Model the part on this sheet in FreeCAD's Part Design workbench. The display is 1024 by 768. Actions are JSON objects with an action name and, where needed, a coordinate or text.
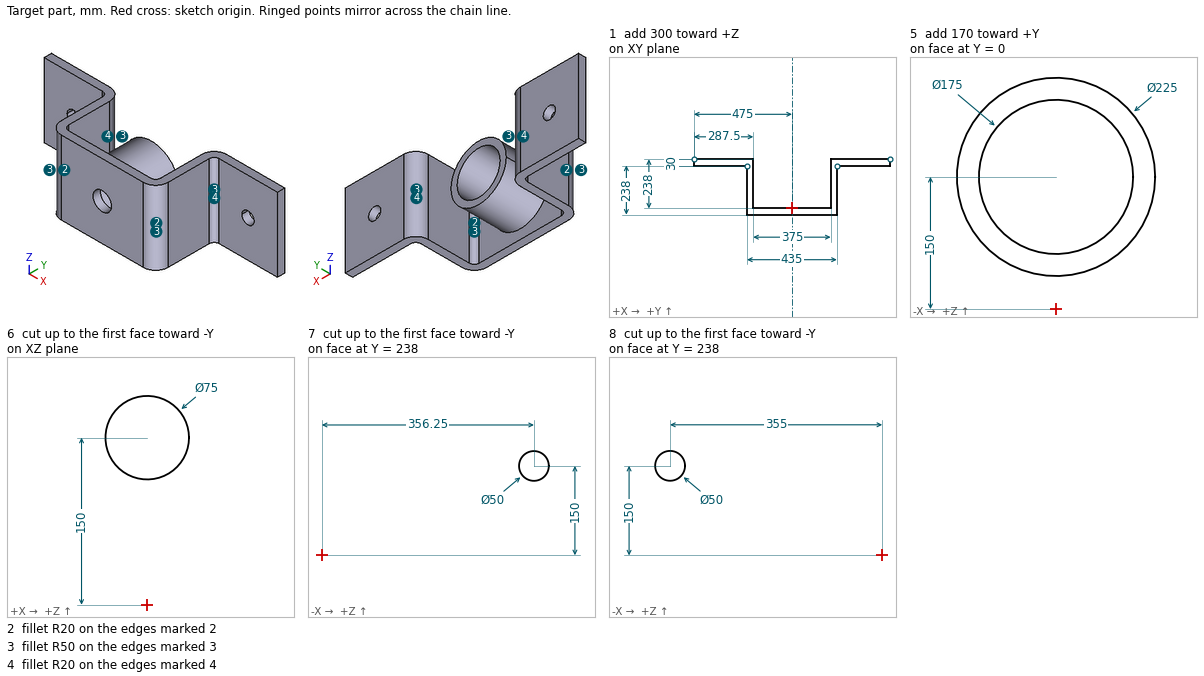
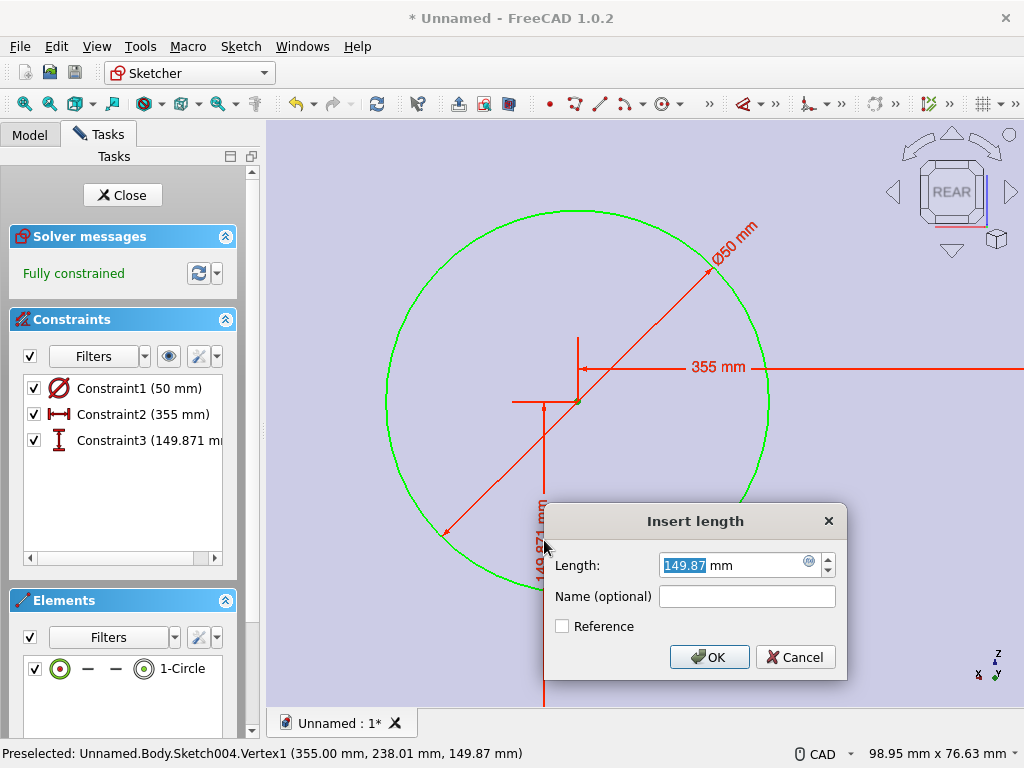
{"action": "type", "text": "150"}
{"action": "key", "text": "Return"}
{"action": "key", "text": "Escape"}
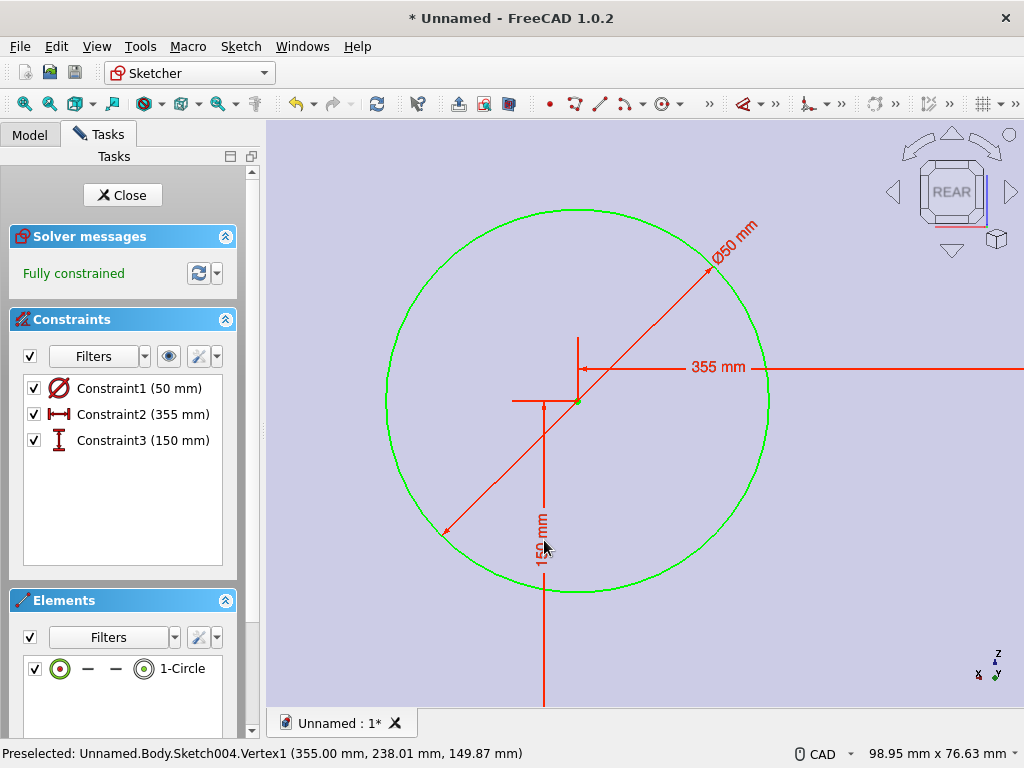
{"action": "left_click", "coordinate": [123, 195]}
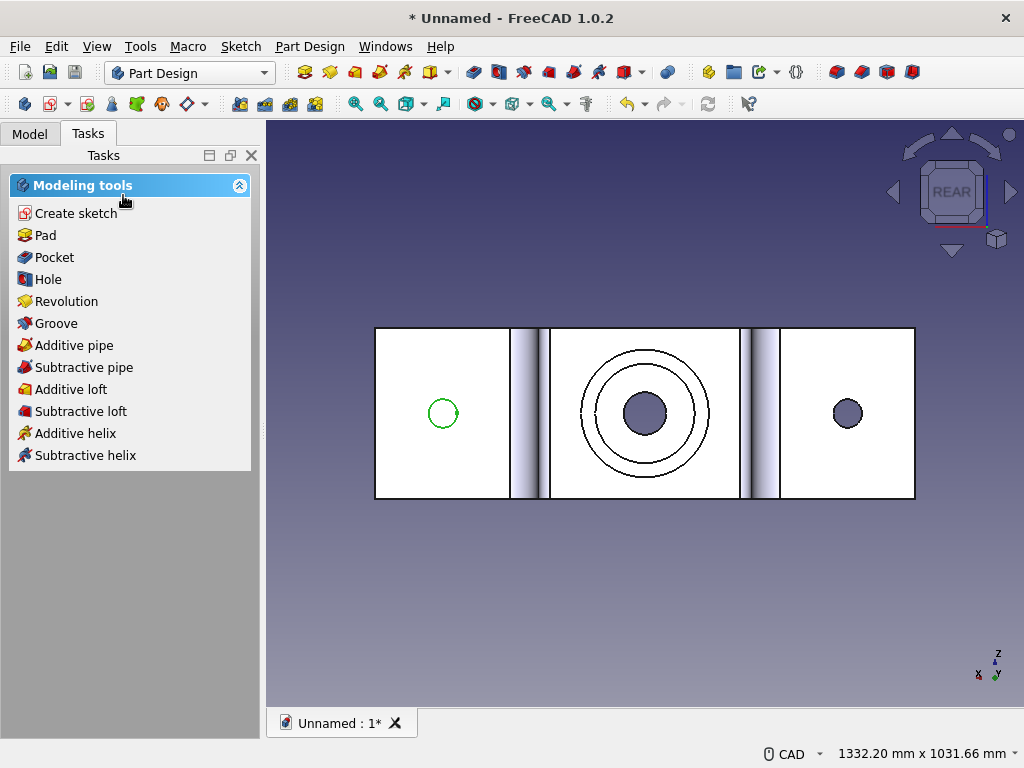
{"action": "left_click", "coordinate": [474, 72]}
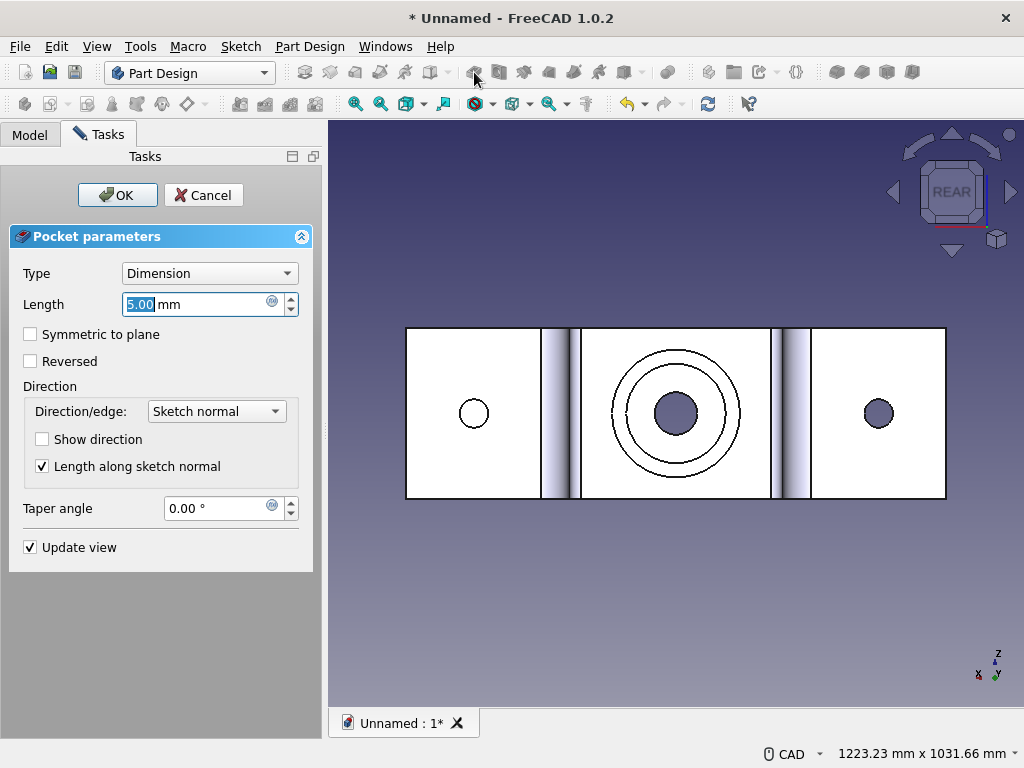
{"action": "left_click", "coordinate": [210, 274]}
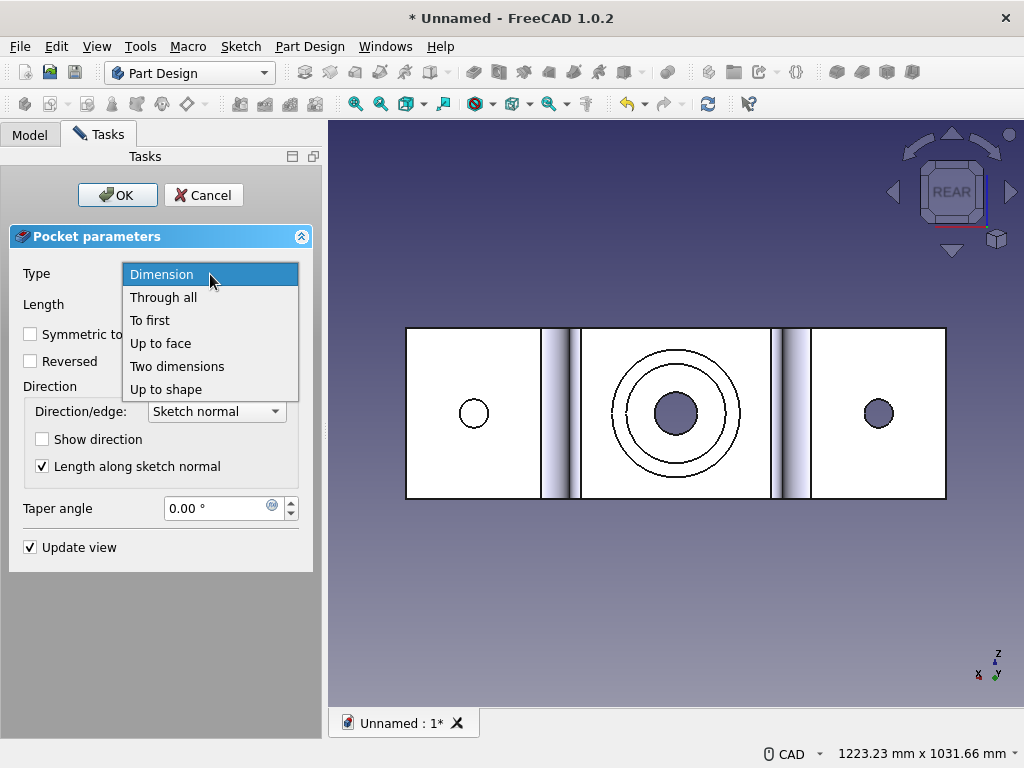
{"action": "left_click", "coordinate": [208, 320]}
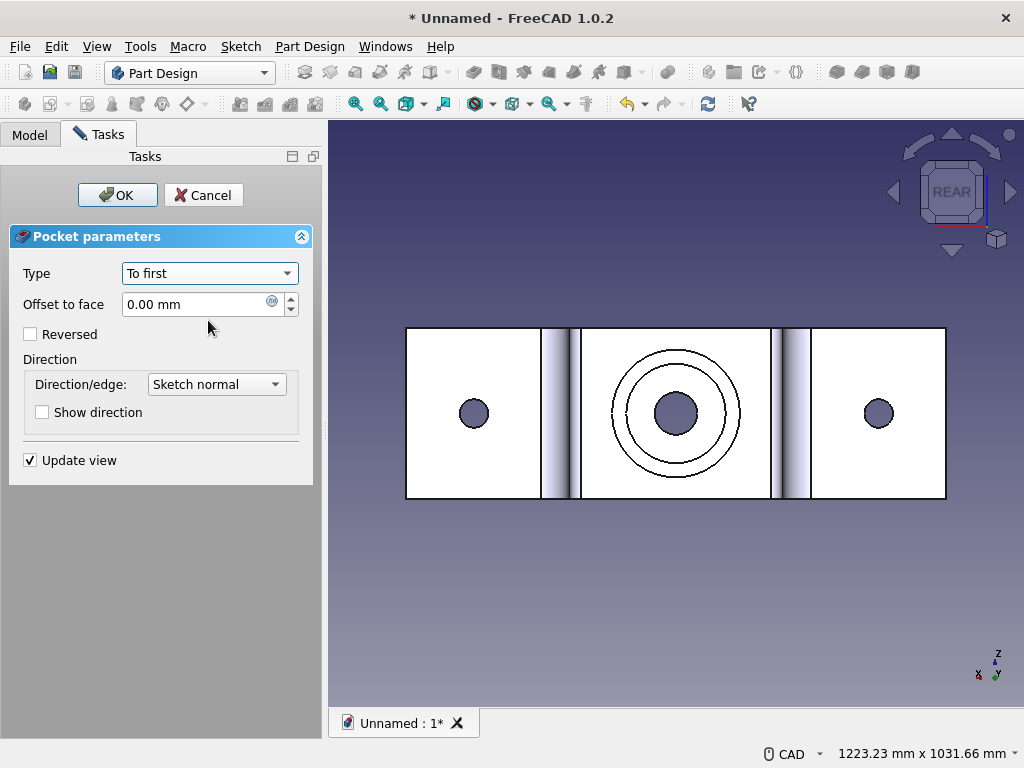
{"action": "left_click", "coordinate": [118, 195]}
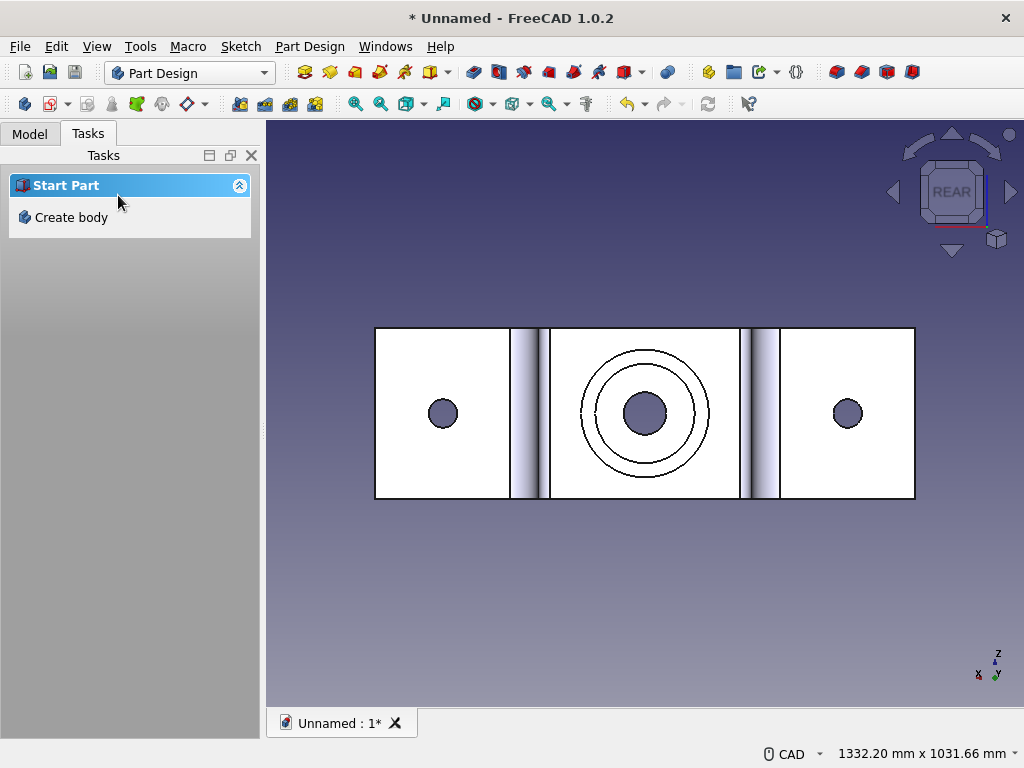
{"action": "key", "text": "0"}